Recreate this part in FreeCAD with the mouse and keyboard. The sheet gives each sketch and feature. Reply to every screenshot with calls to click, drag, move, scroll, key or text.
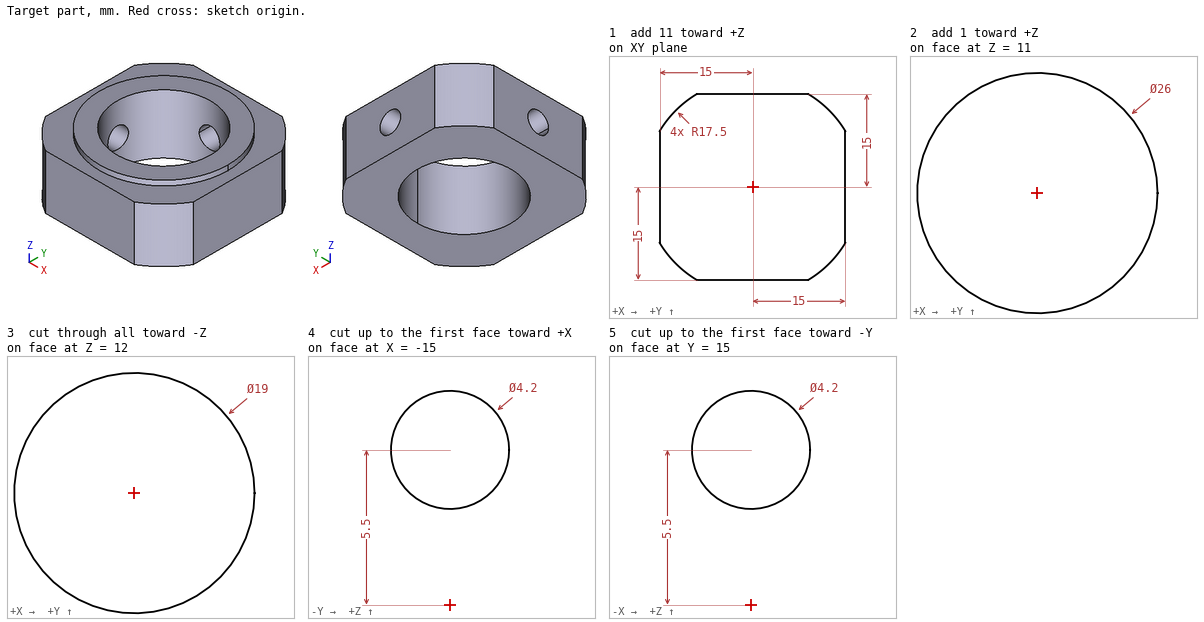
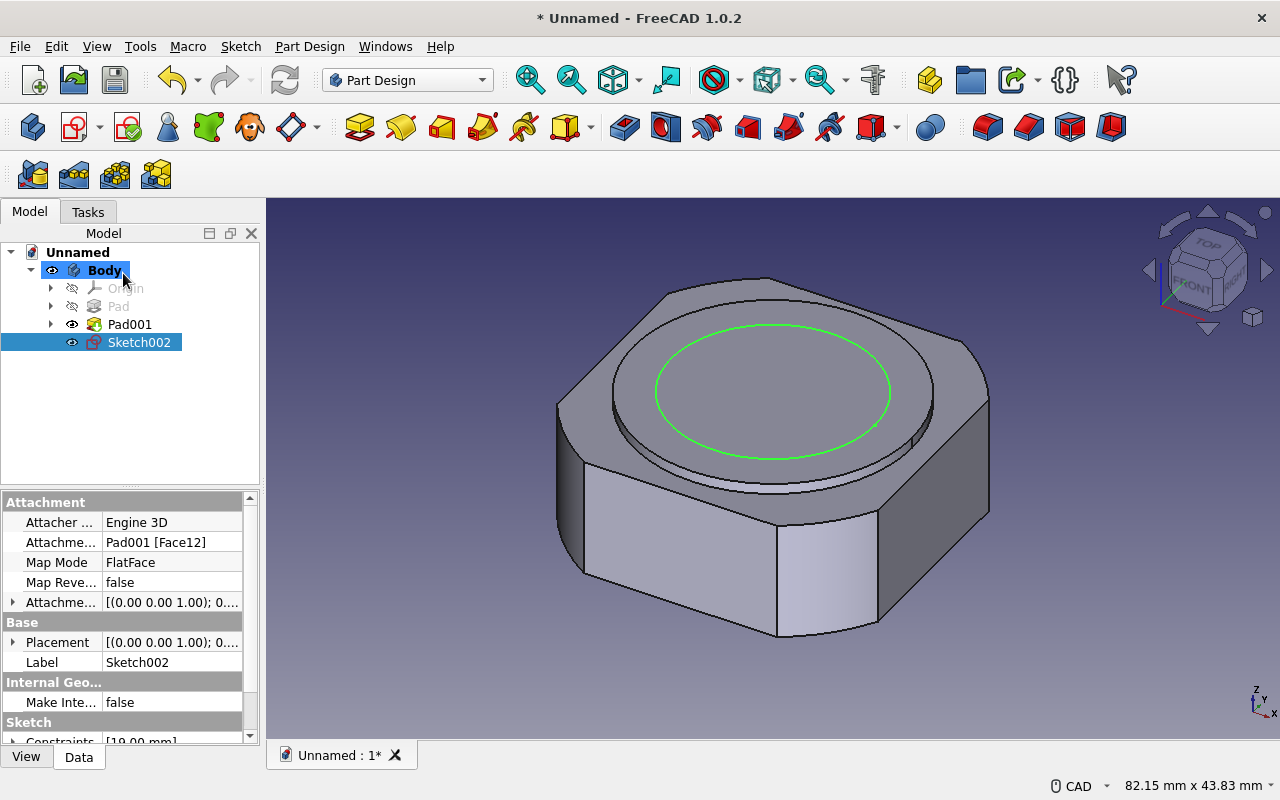
click(625, 128)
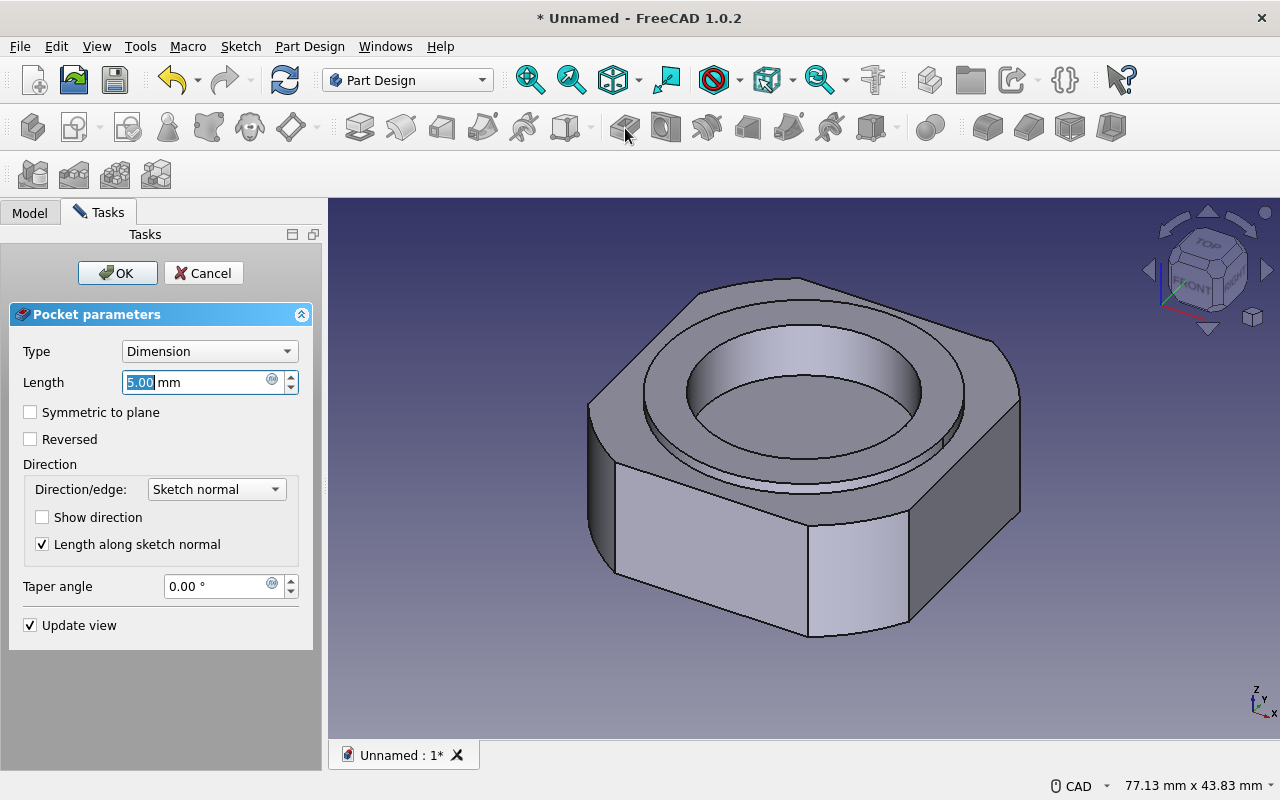
click(210, 352)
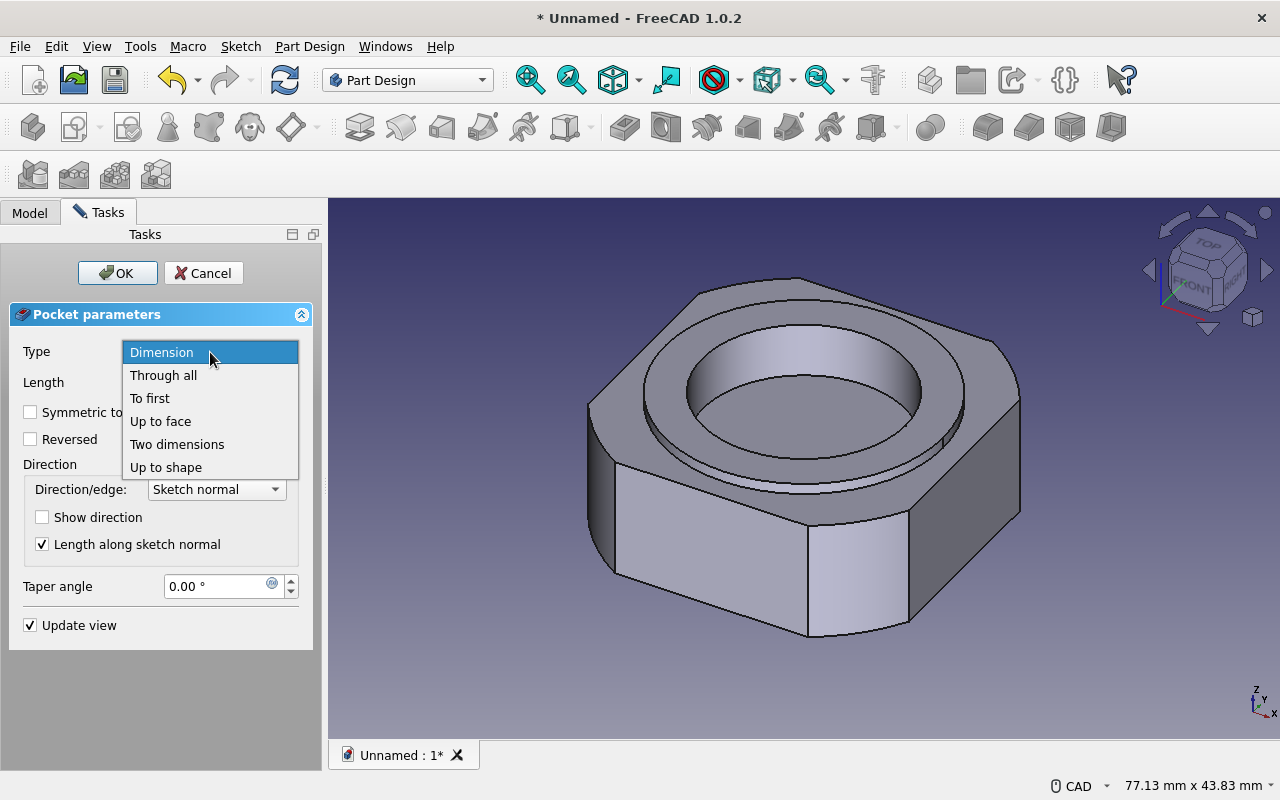
click(208, 376)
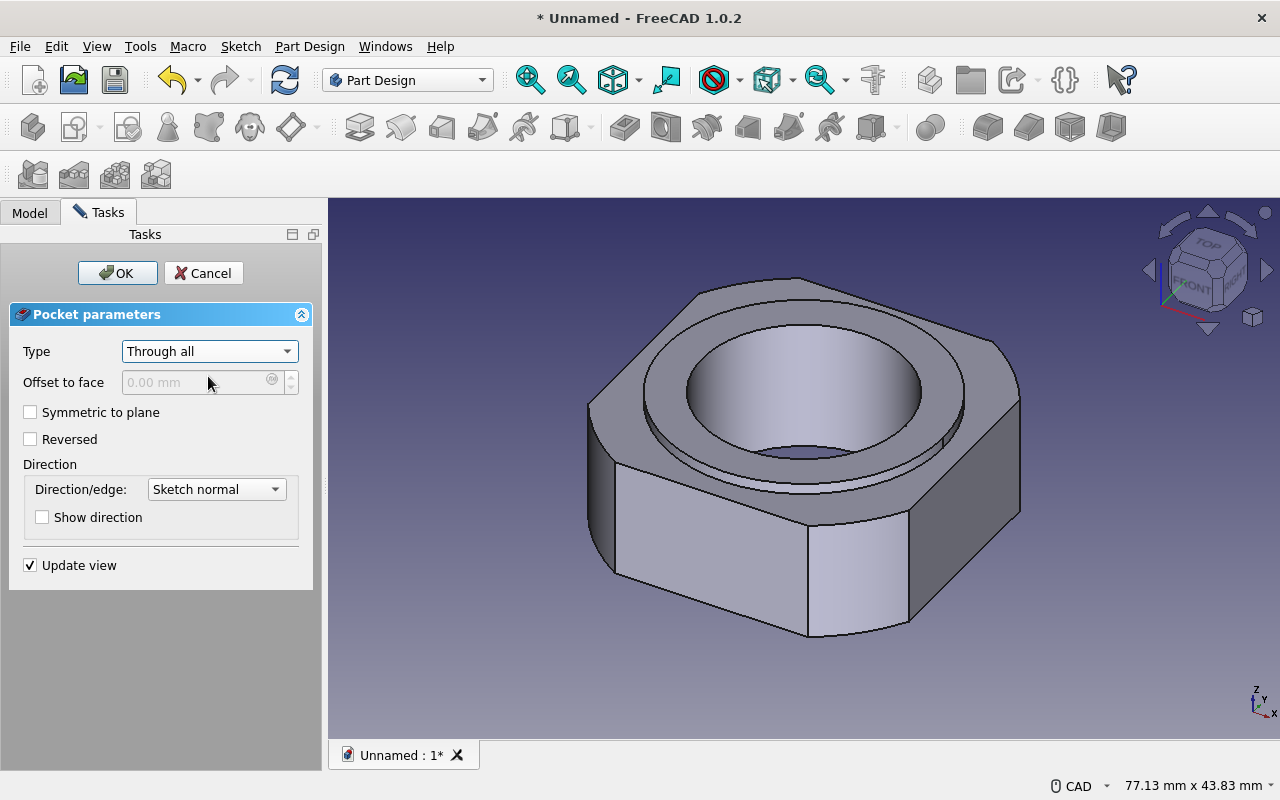
click(118, 273)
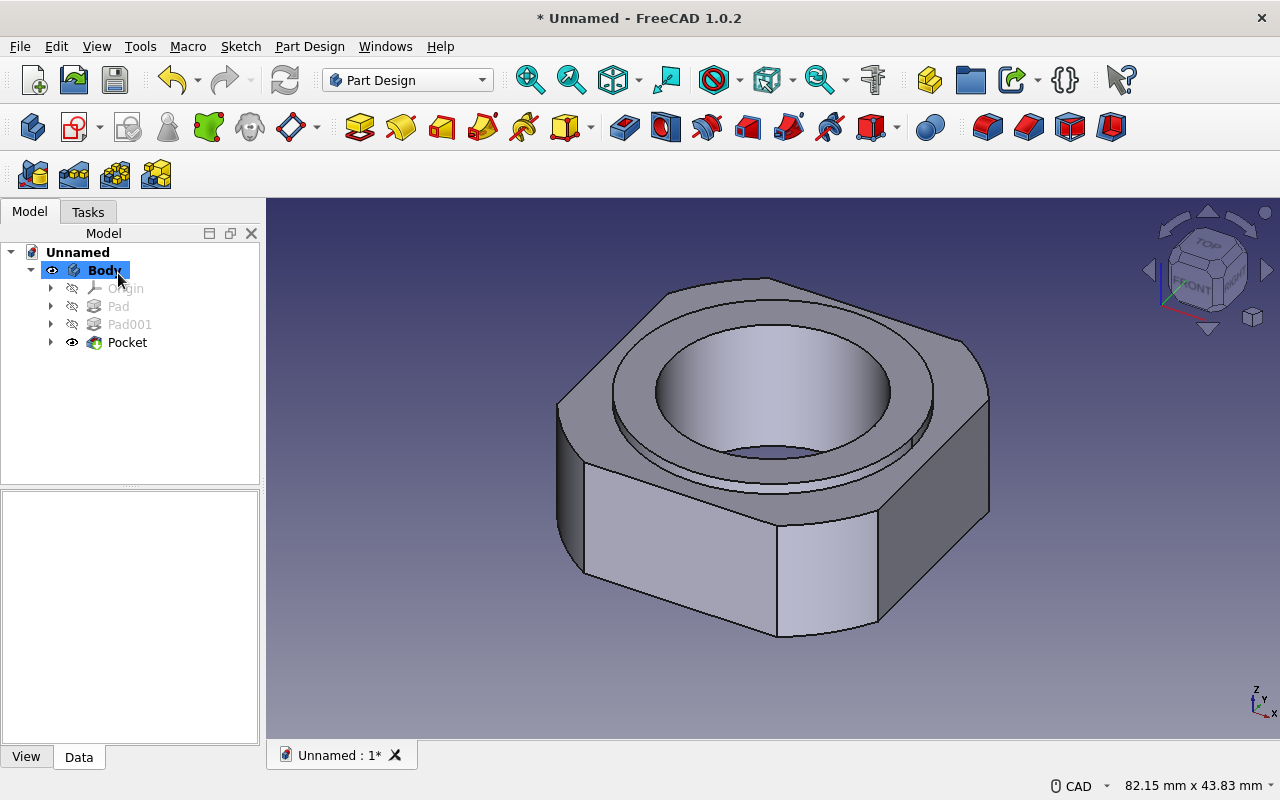
key(6)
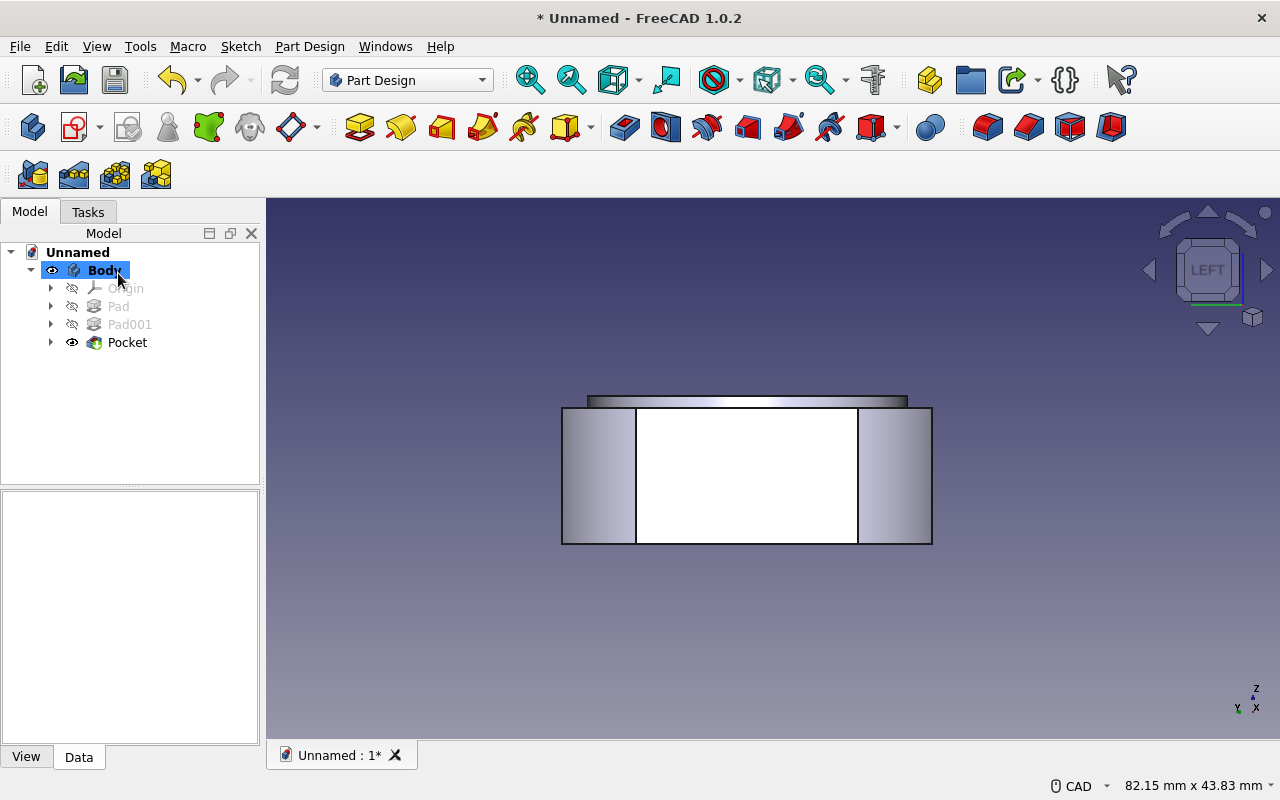
click(531, 80)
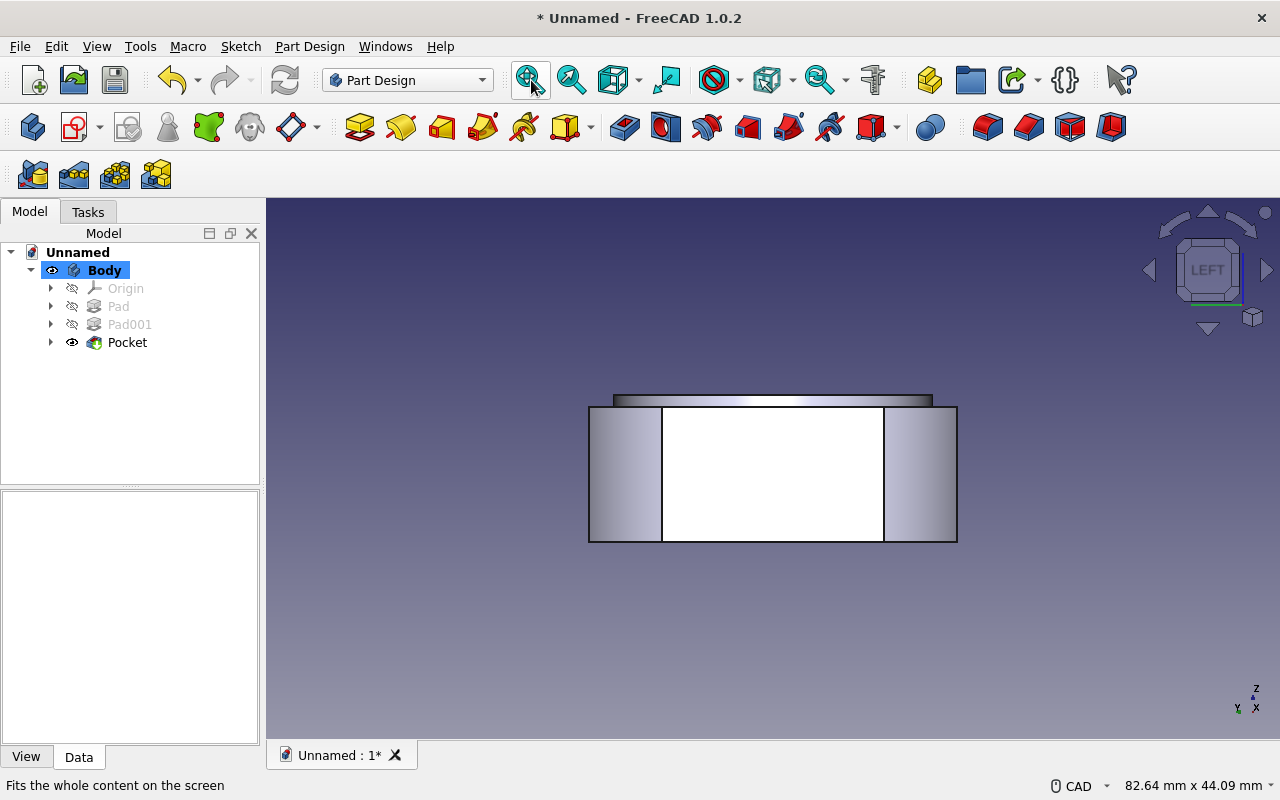
click(741, 474)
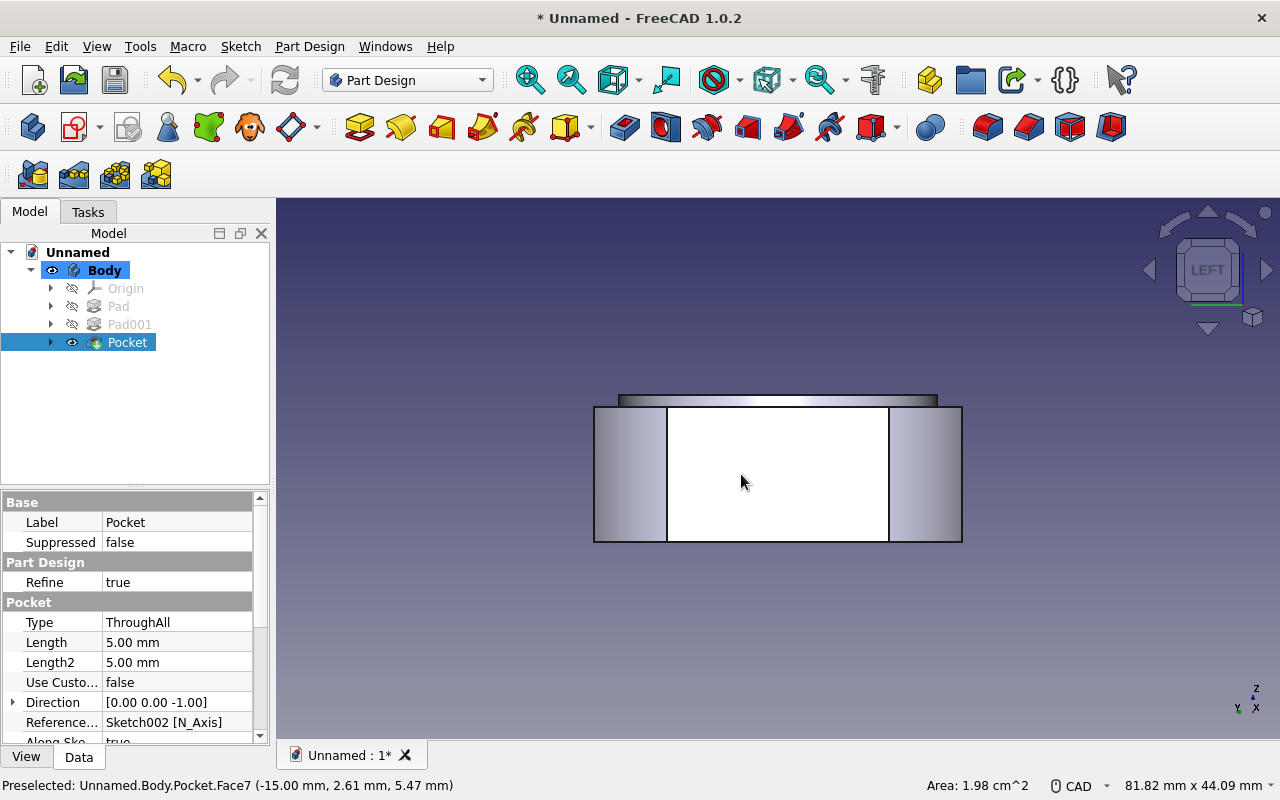
click(74, 128)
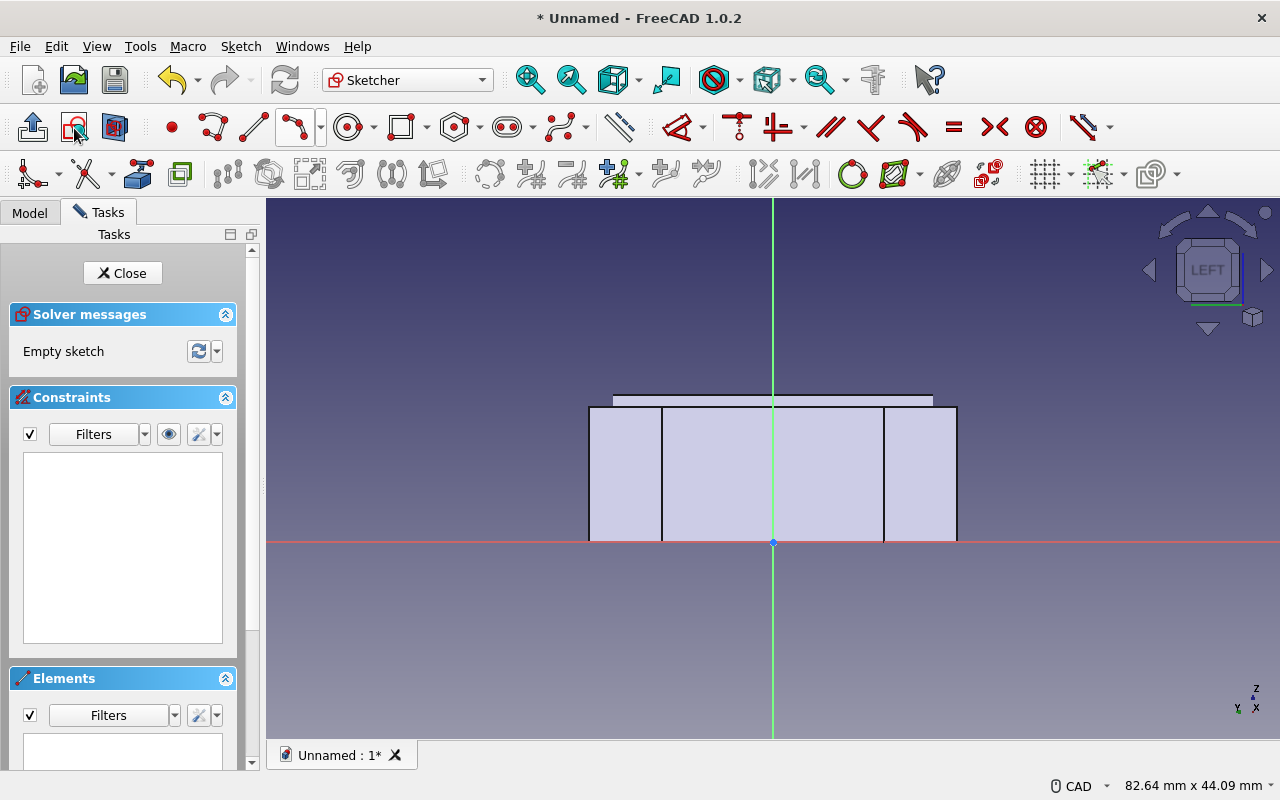
scroll(795, 504, up, 7)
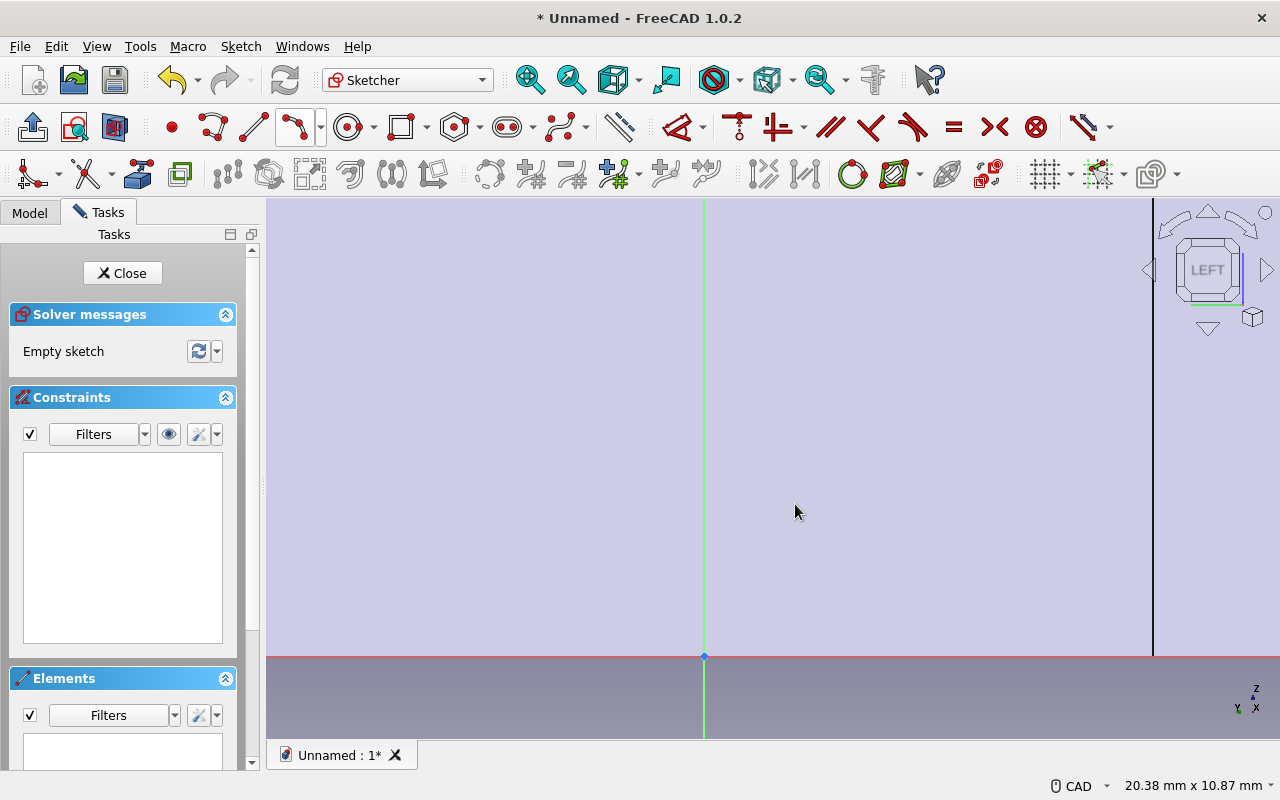
click(348, 128)